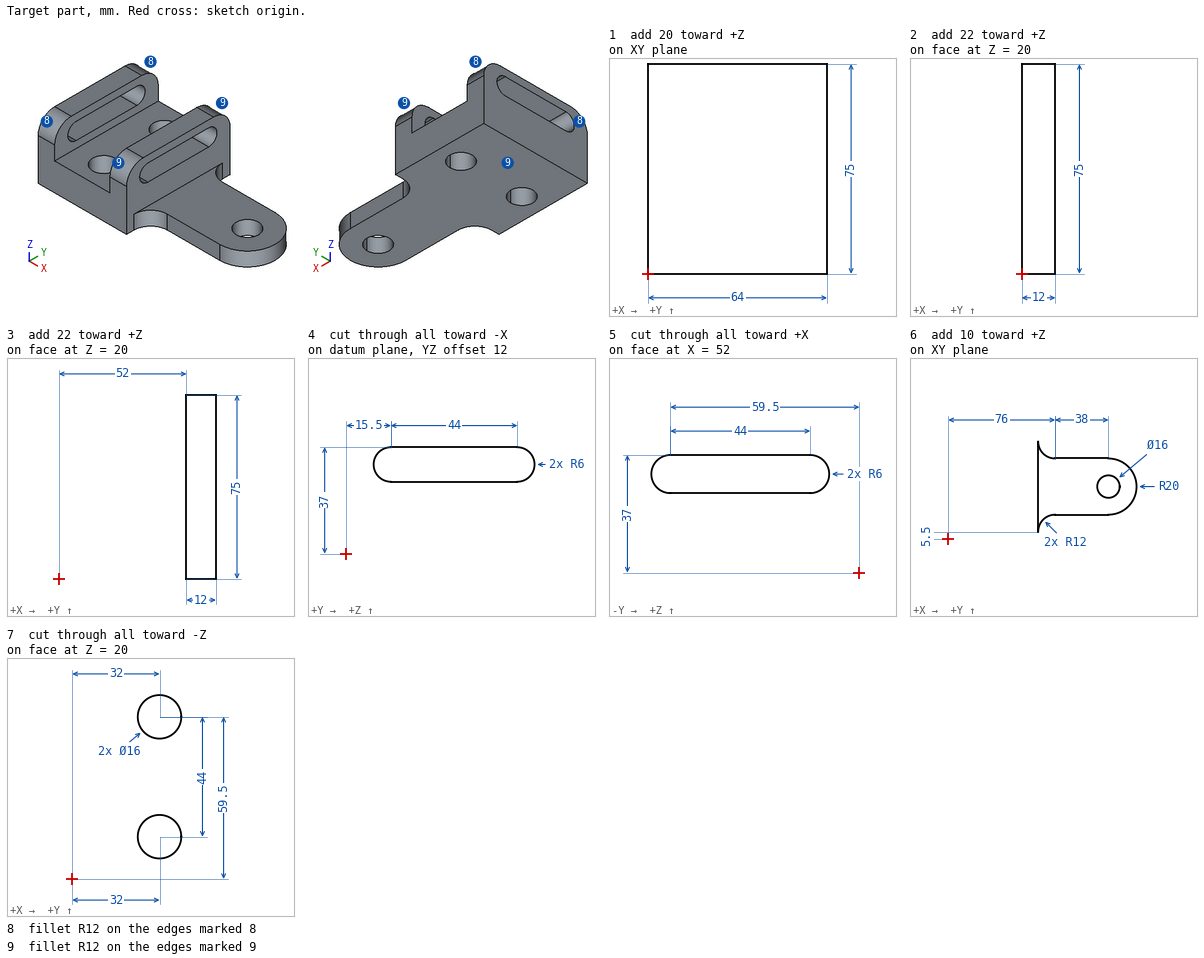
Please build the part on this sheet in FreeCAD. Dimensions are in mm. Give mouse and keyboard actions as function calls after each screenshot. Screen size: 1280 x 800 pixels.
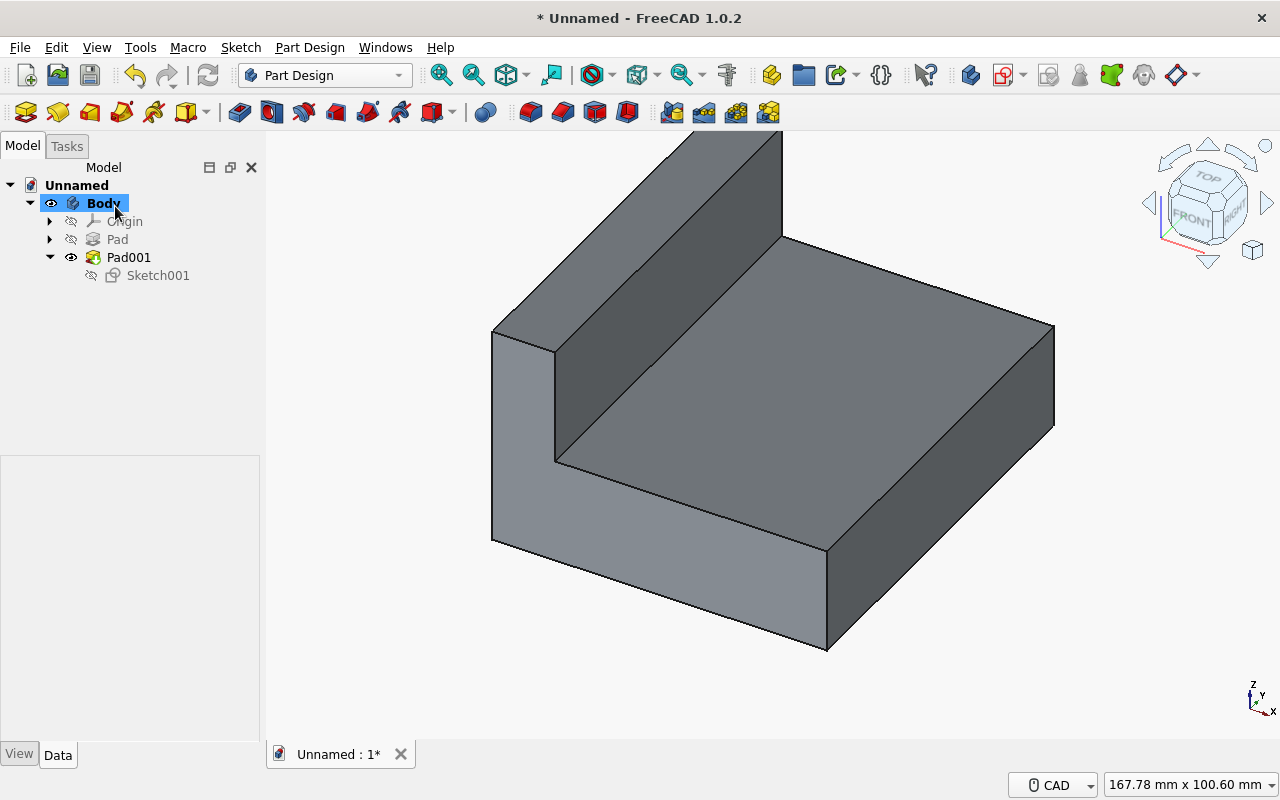
click(442, 76)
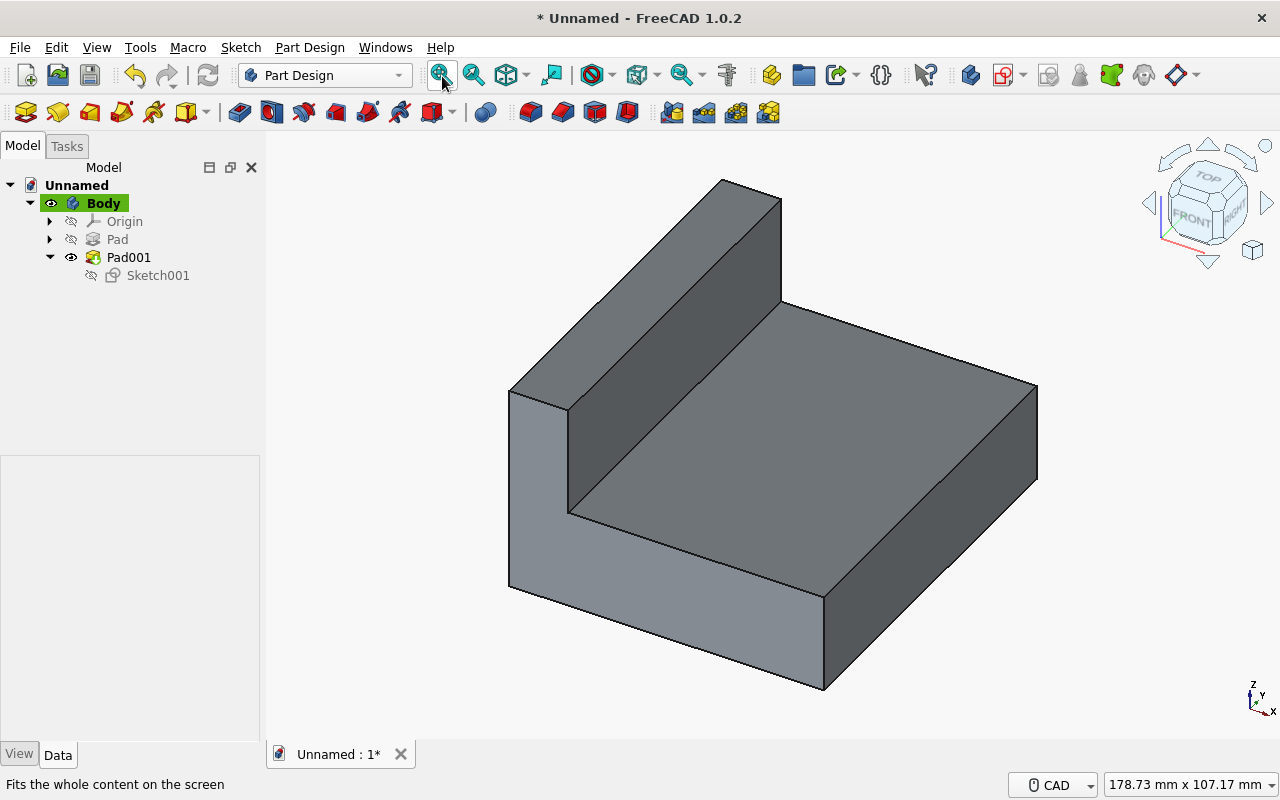
click(833, 418)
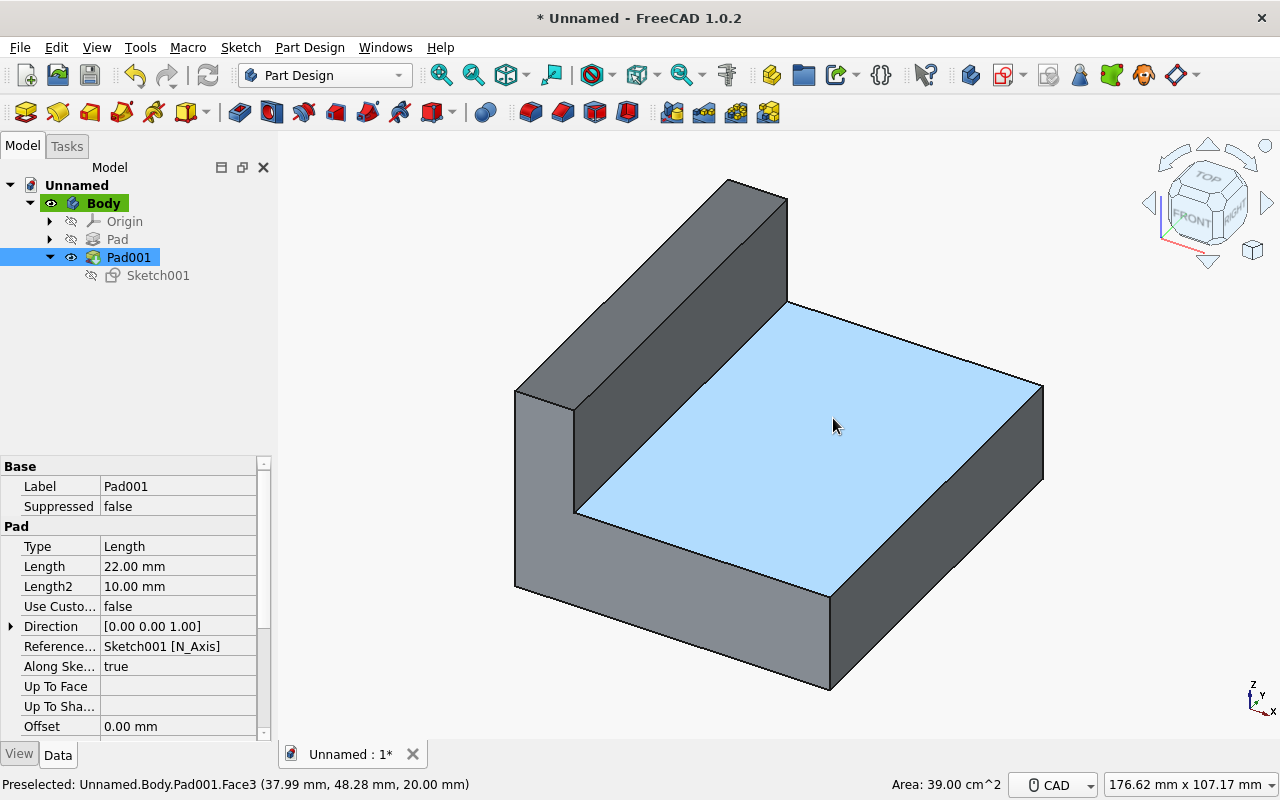
click(1004, 76)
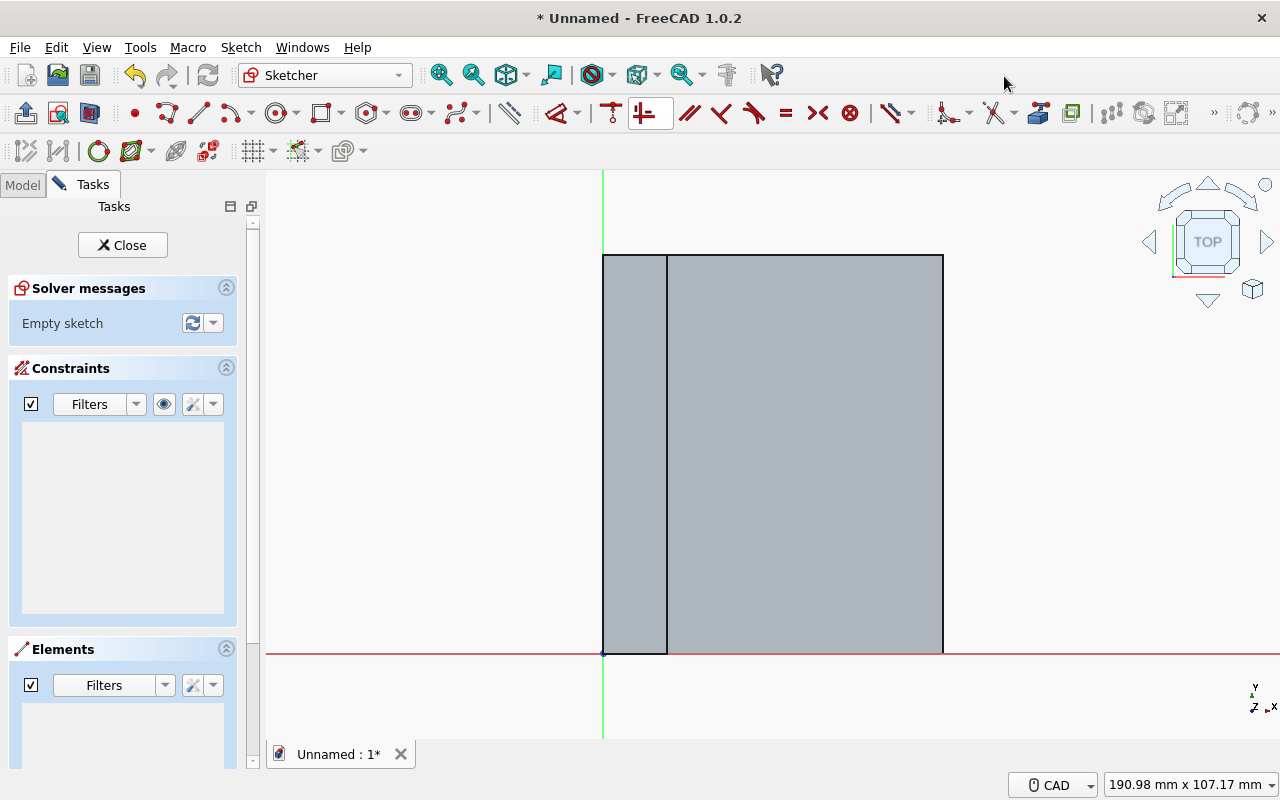
click(322, 114)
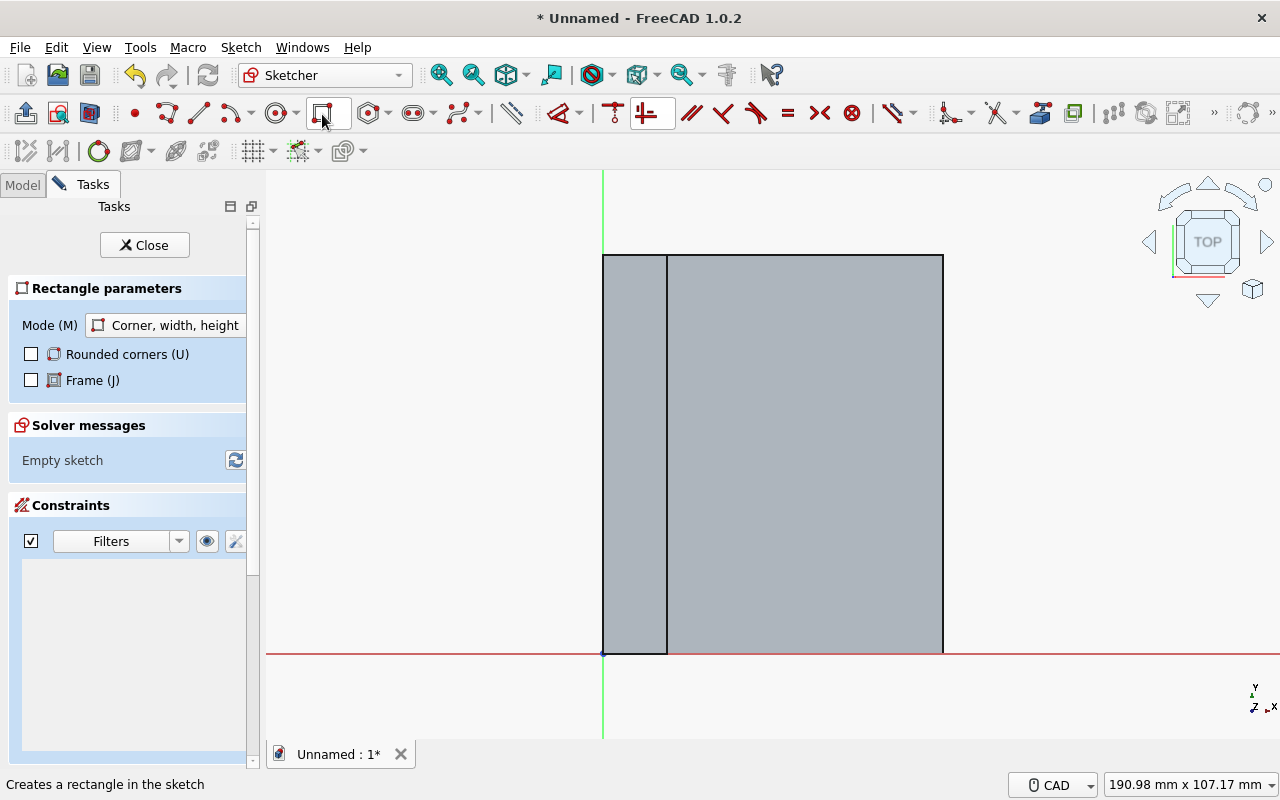
click(879, 255)
click(943, 654)
key(Escape)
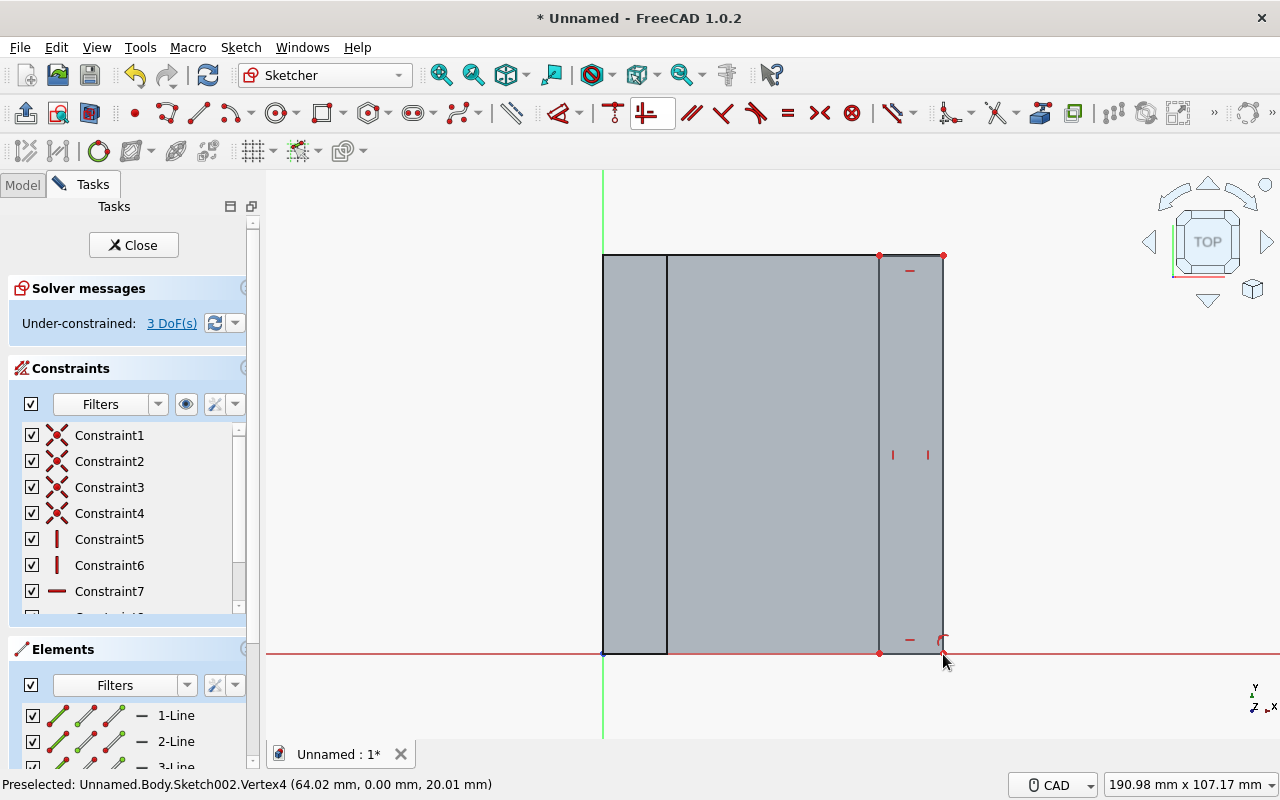
click(558, 114)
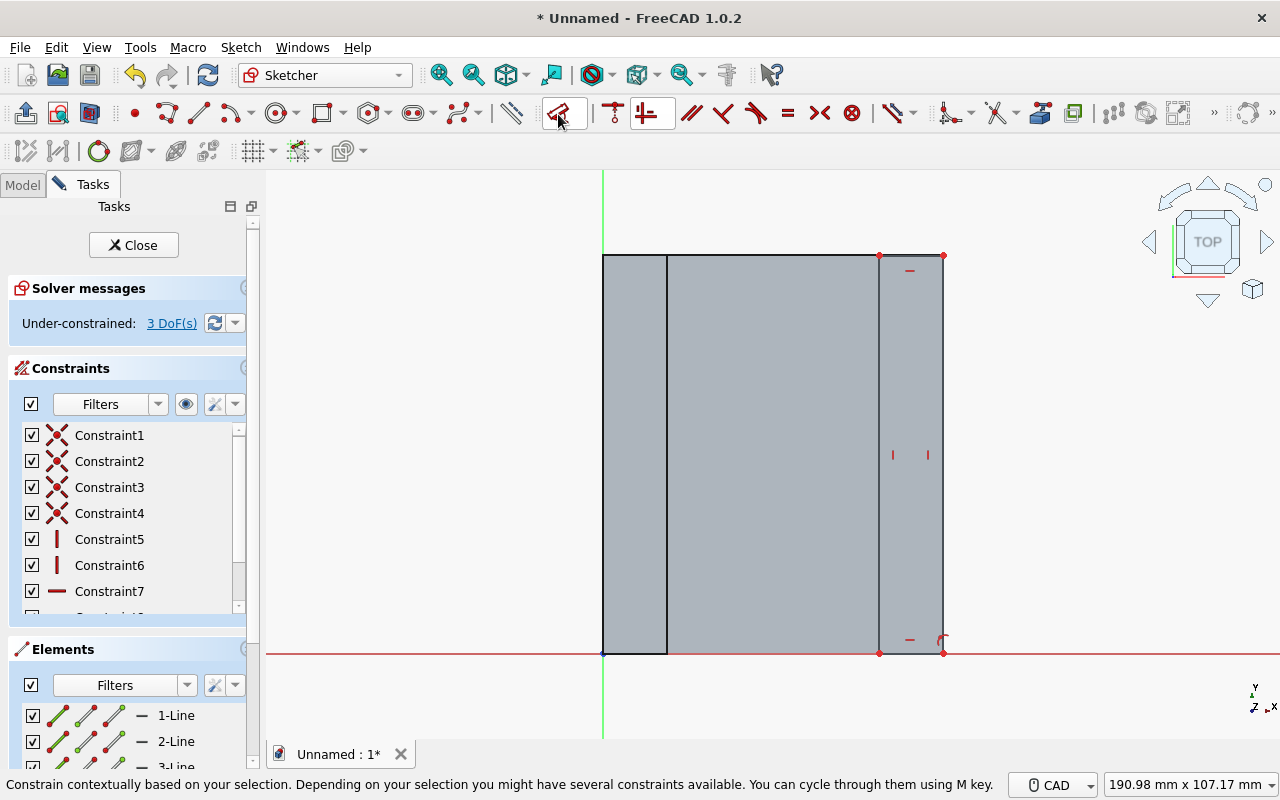
click(879, 375)
click(913, 455)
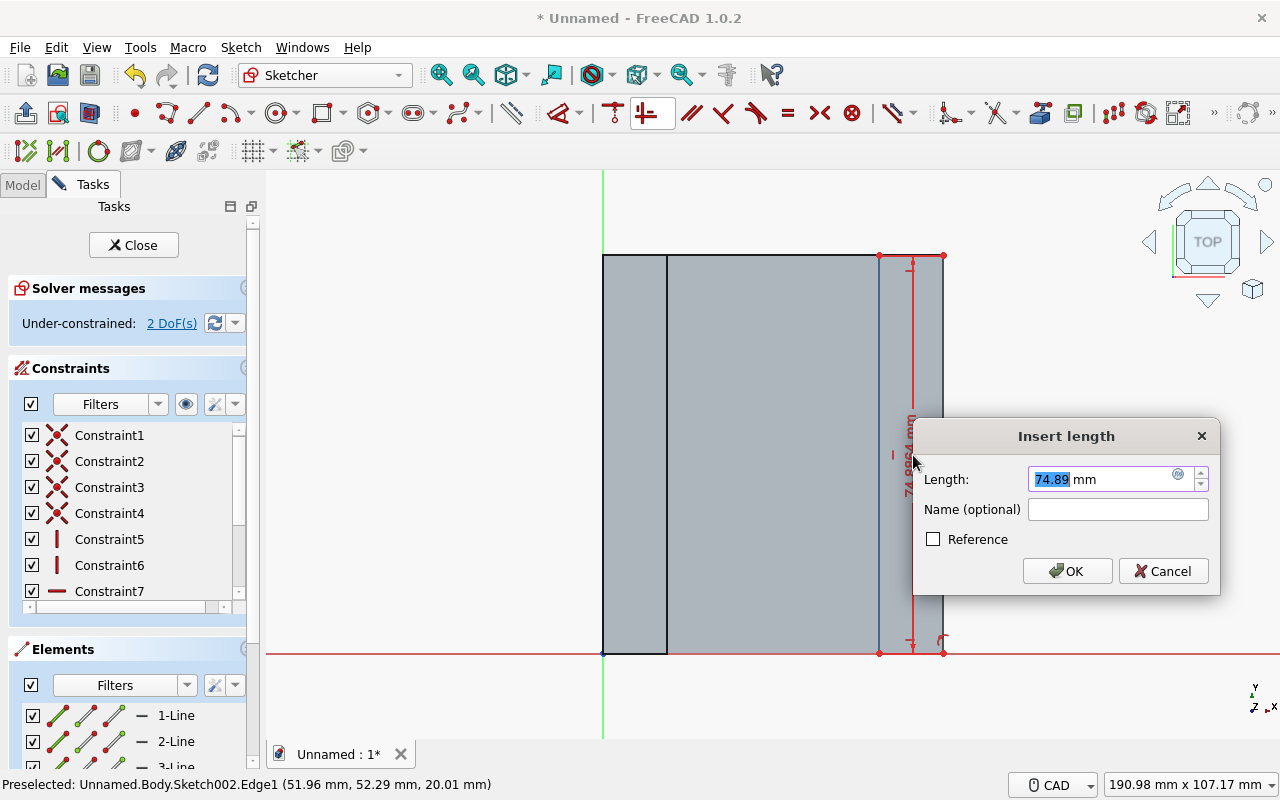
text(75)
key(Return)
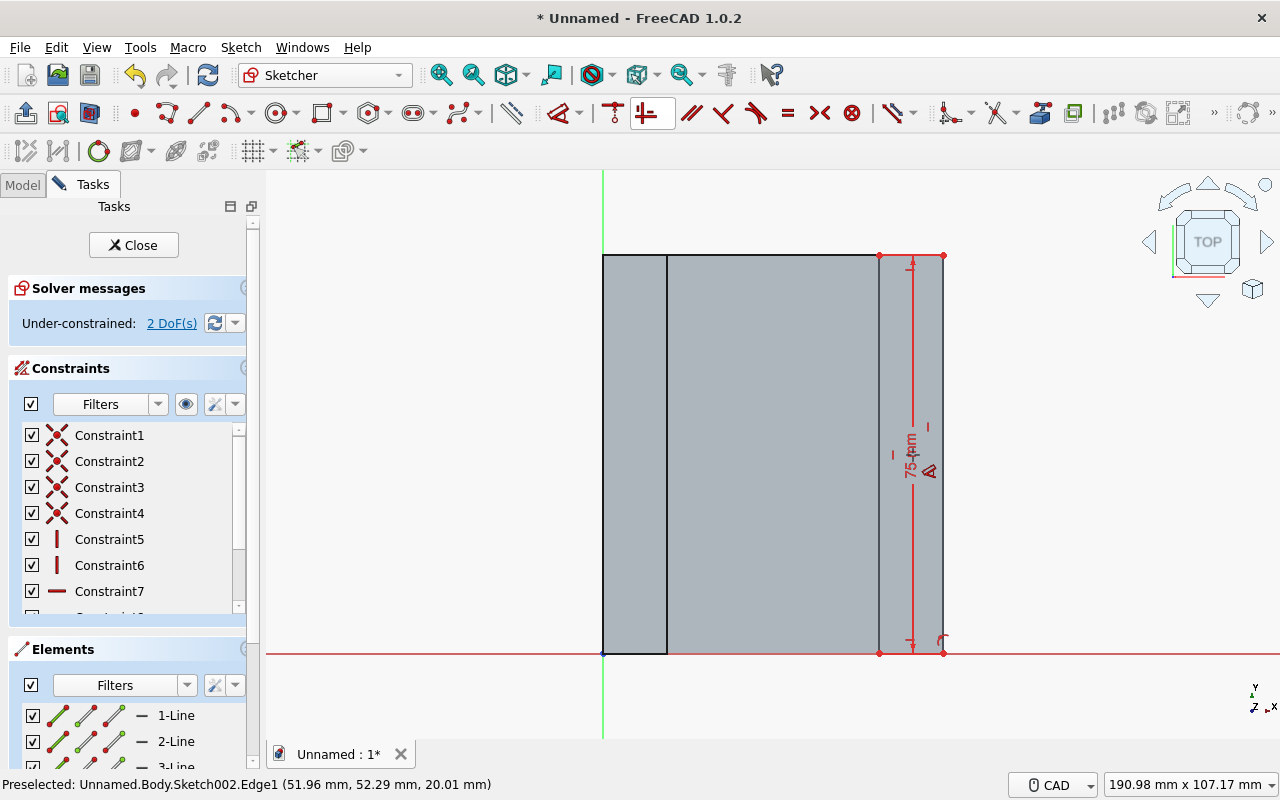
click(898, 654)
click(911, 688)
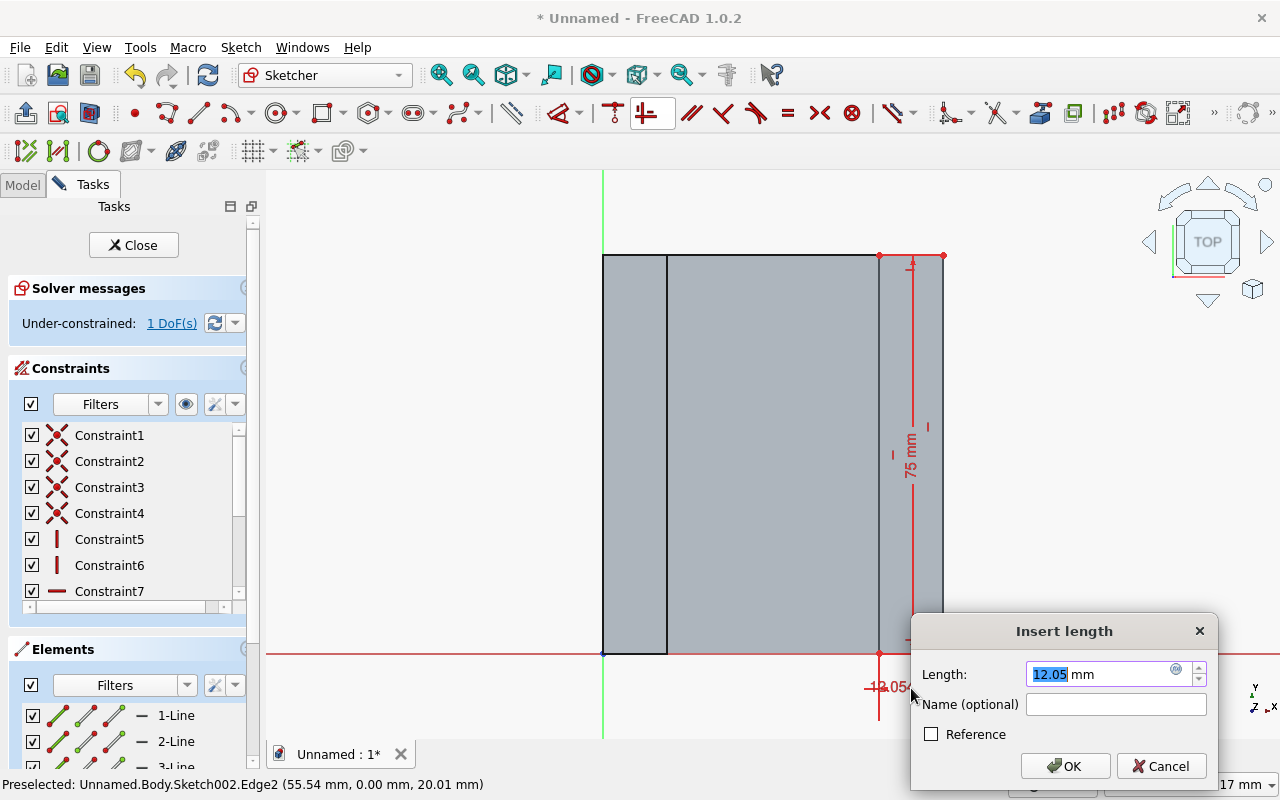
text(12)
key(Return)